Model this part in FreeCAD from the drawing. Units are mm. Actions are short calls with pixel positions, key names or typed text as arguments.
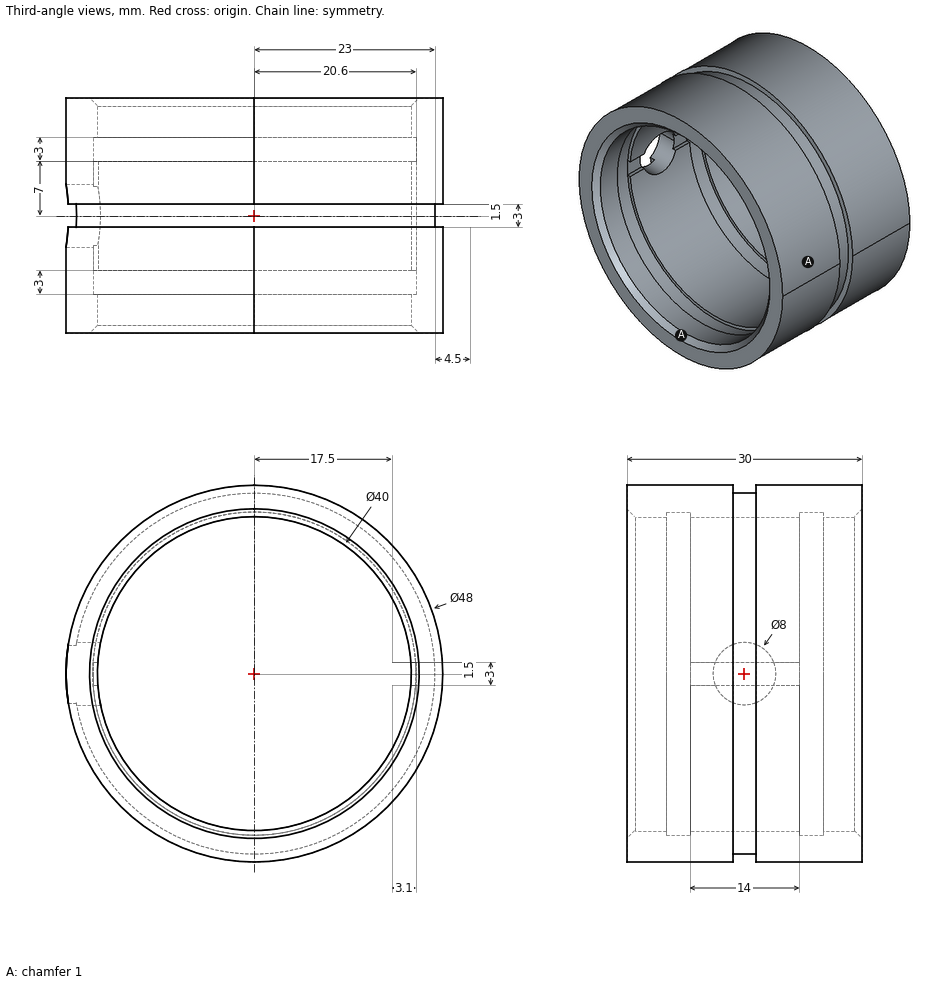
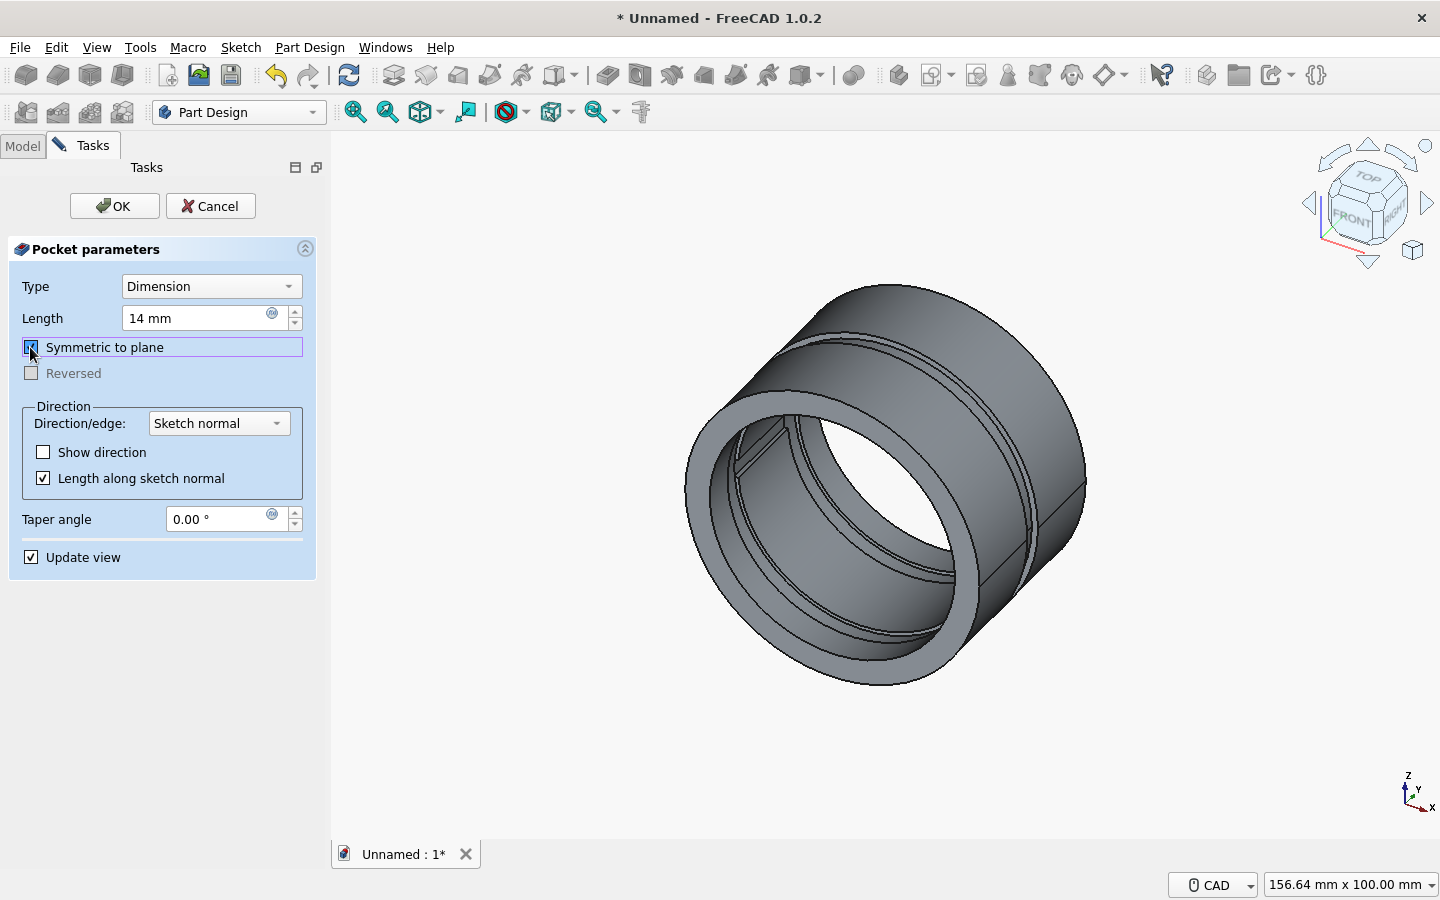
click(115, 206)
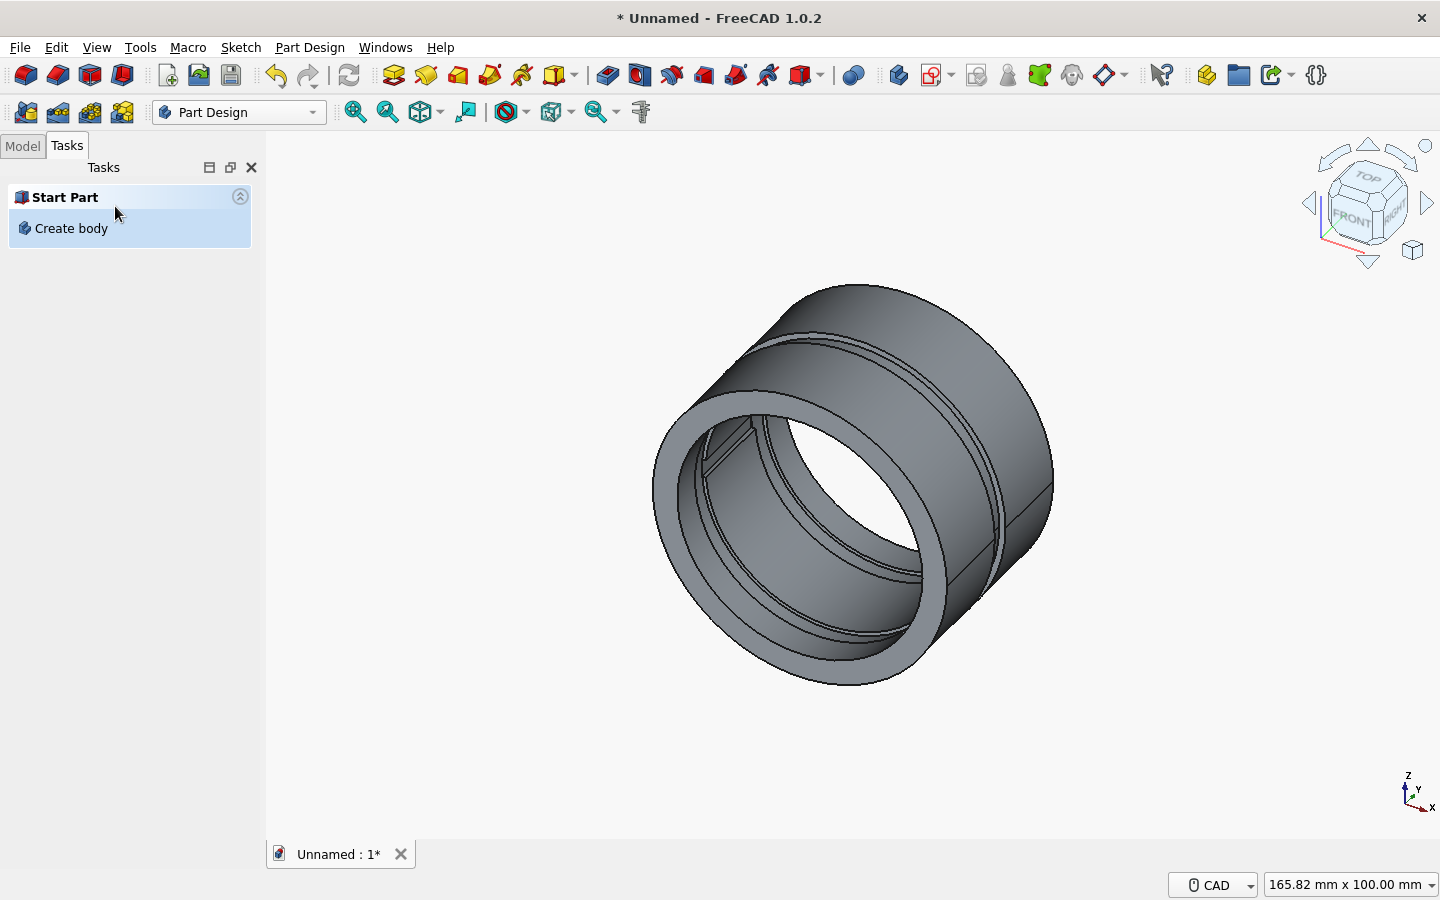
click(932, 76)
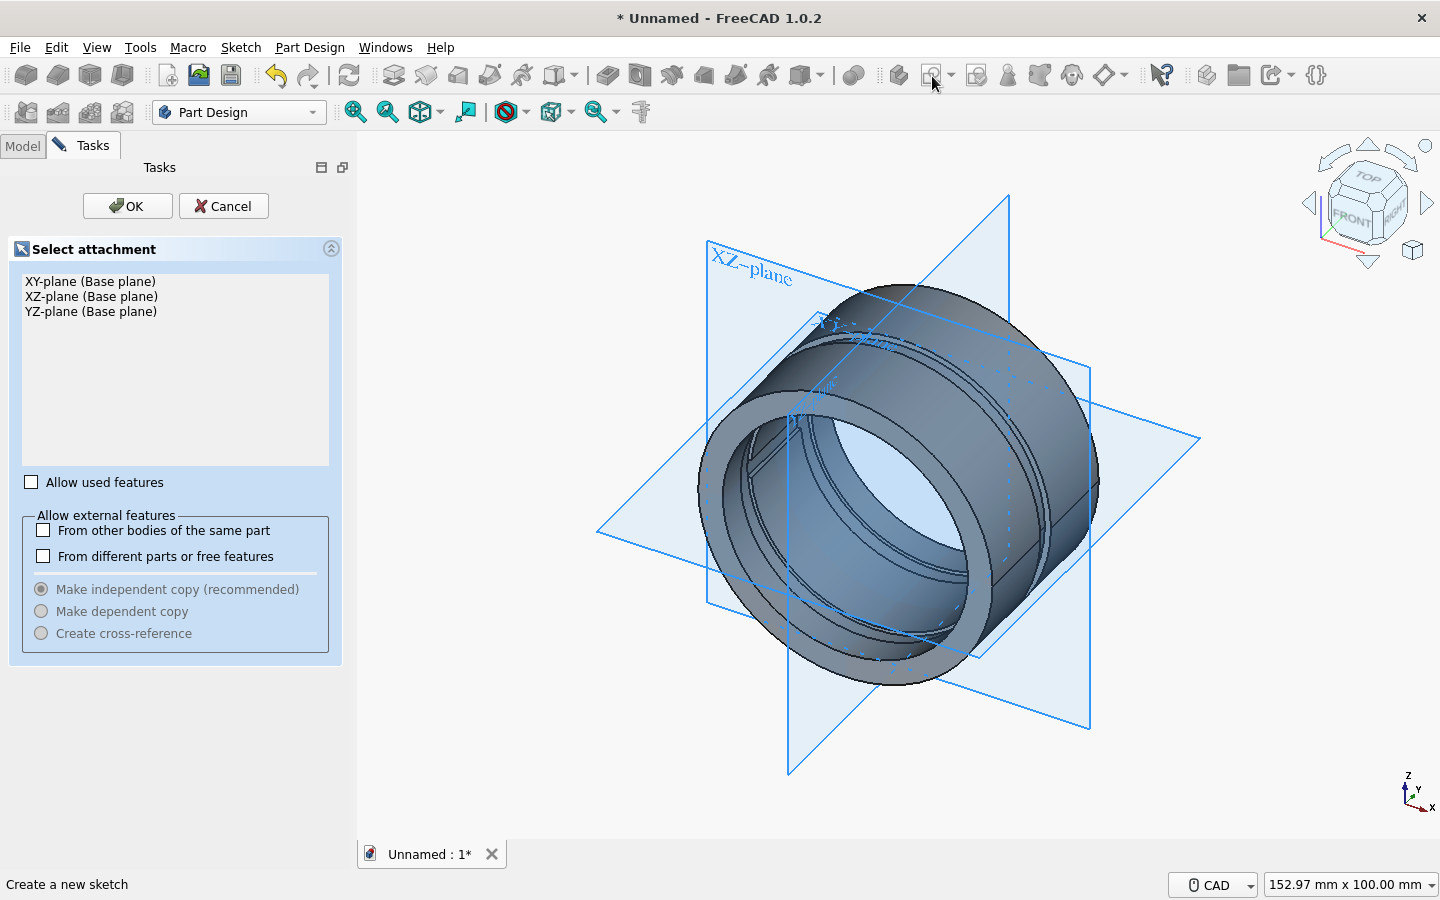
click(82, 312)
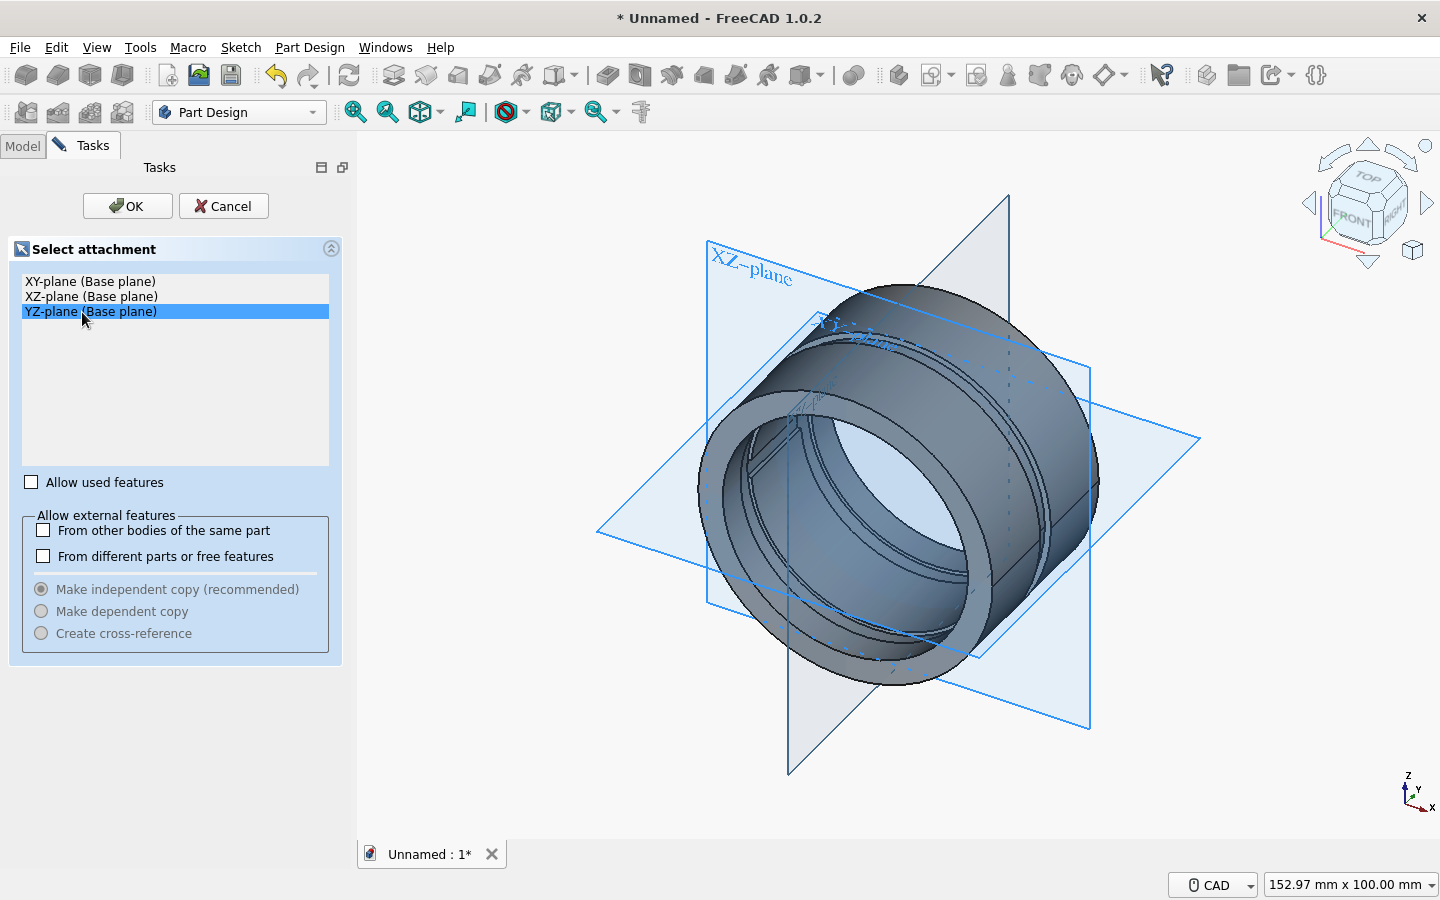
click(128, 206)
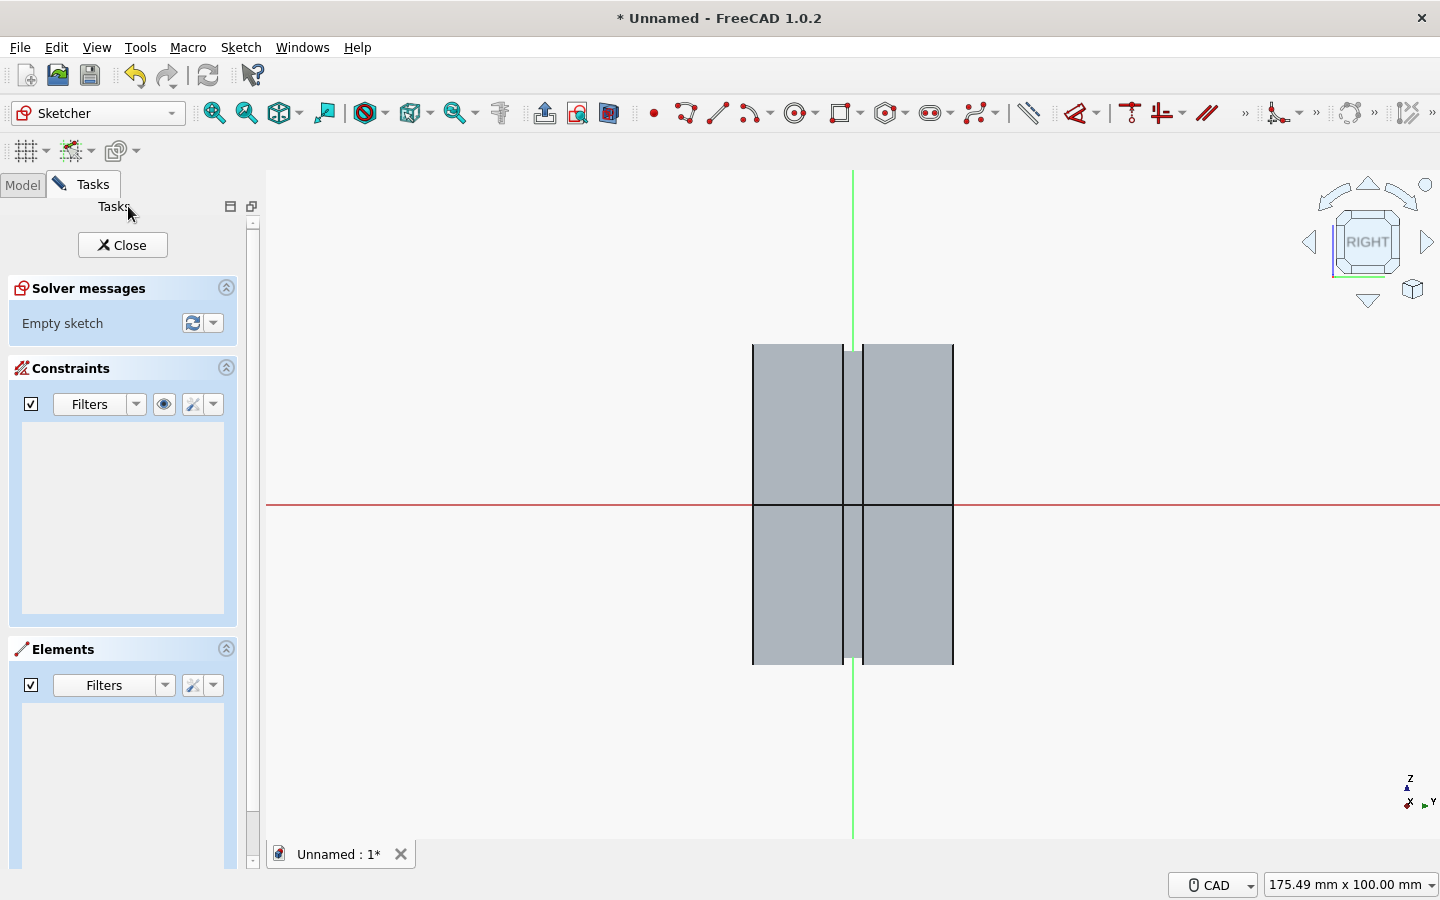
key(q)
key(s)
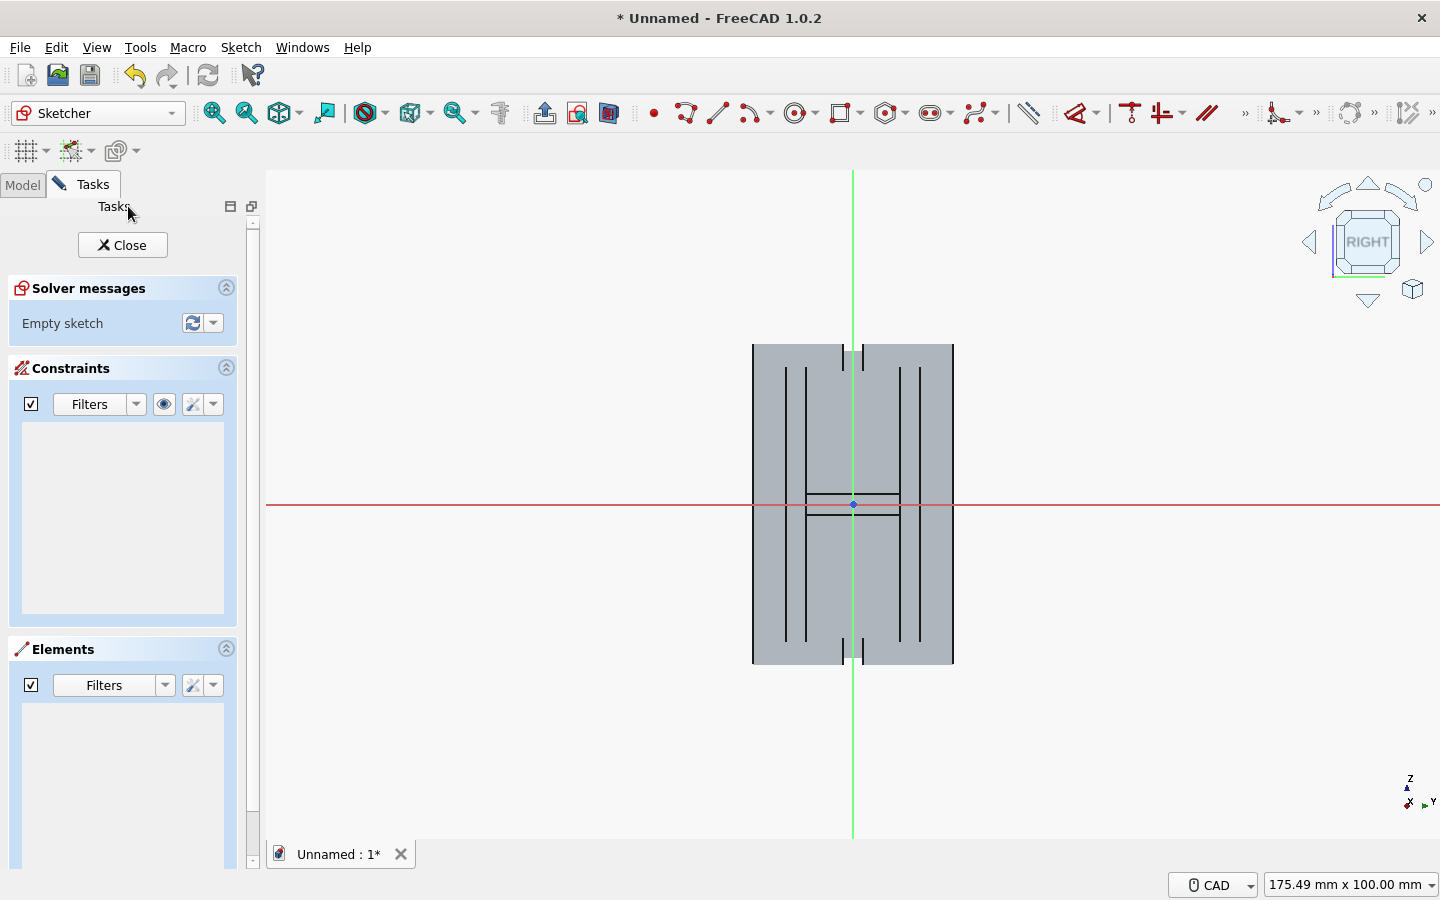
scroll(864, 504, up, 10)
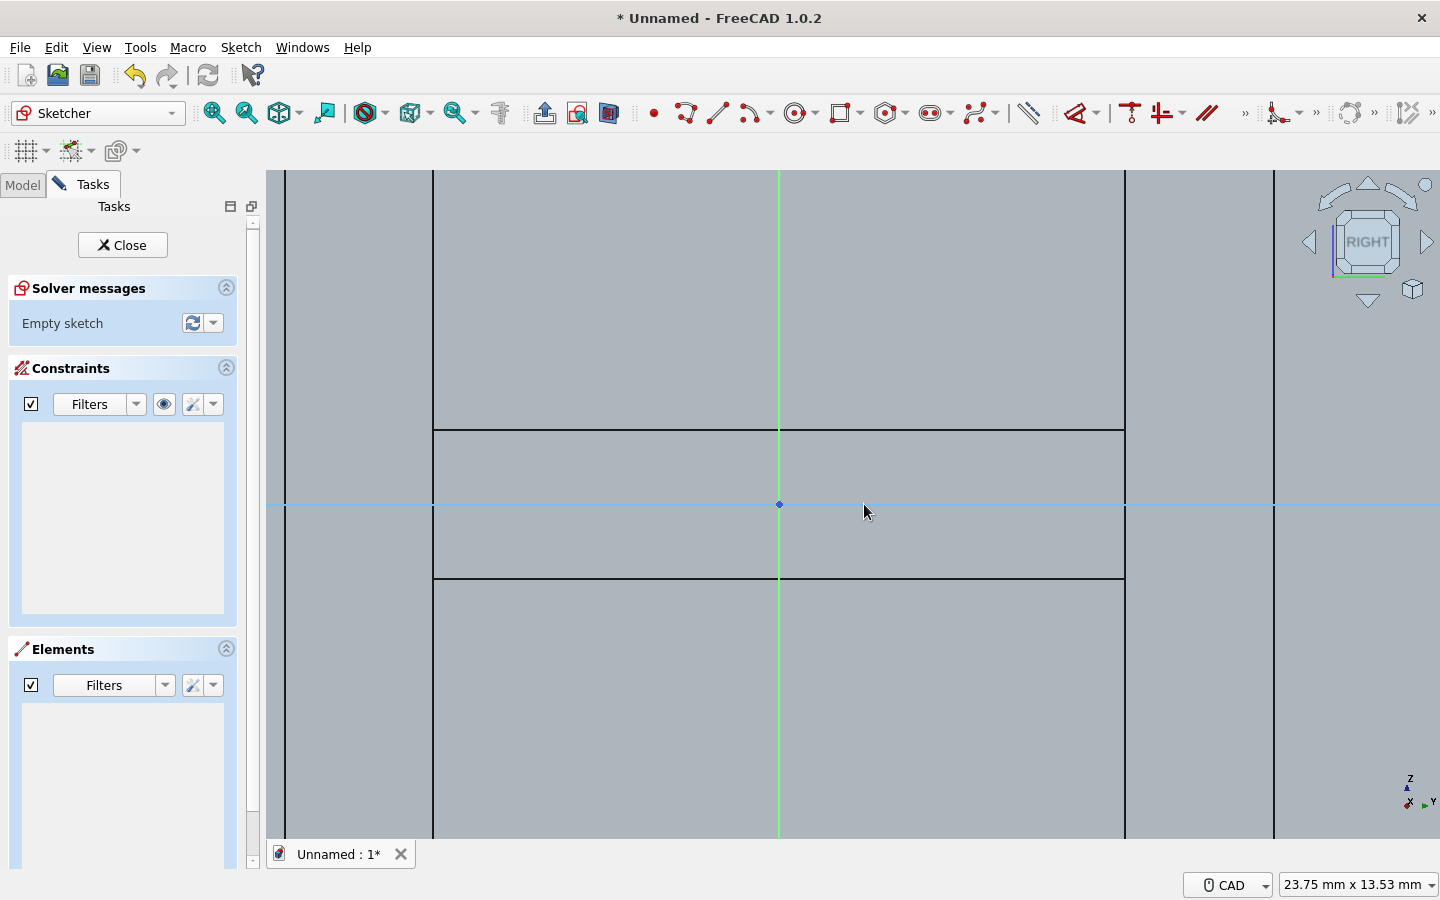
click(796, 114)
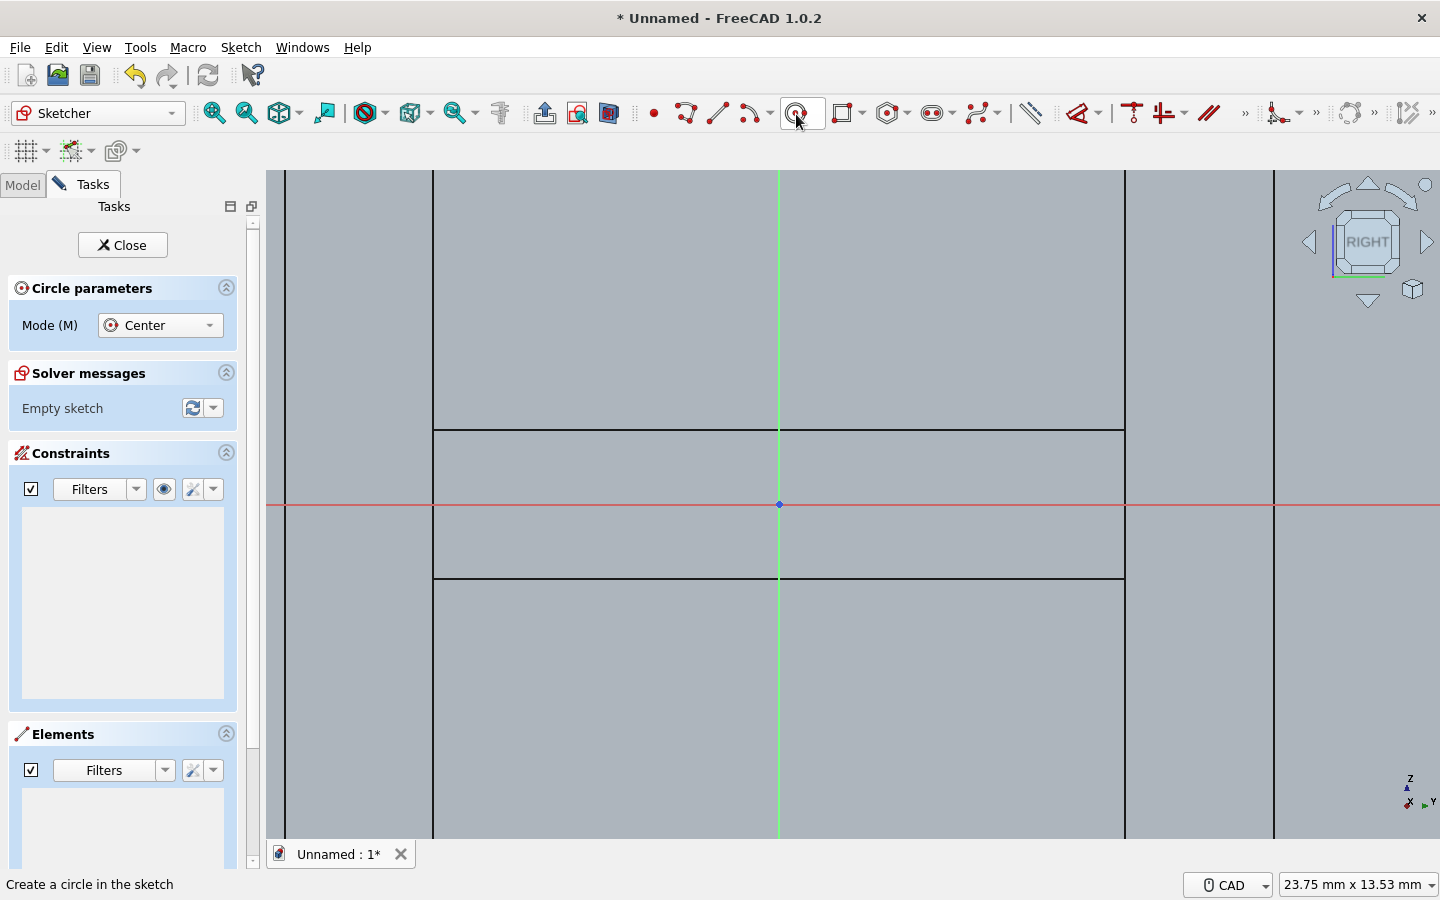
click(779, 504)
click(919, 365)
key(Escape)